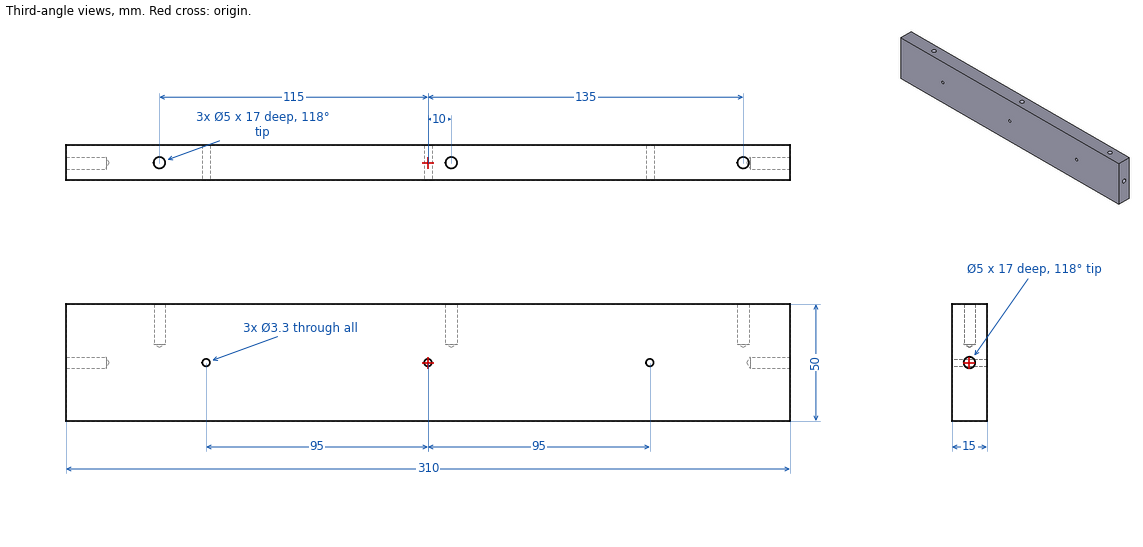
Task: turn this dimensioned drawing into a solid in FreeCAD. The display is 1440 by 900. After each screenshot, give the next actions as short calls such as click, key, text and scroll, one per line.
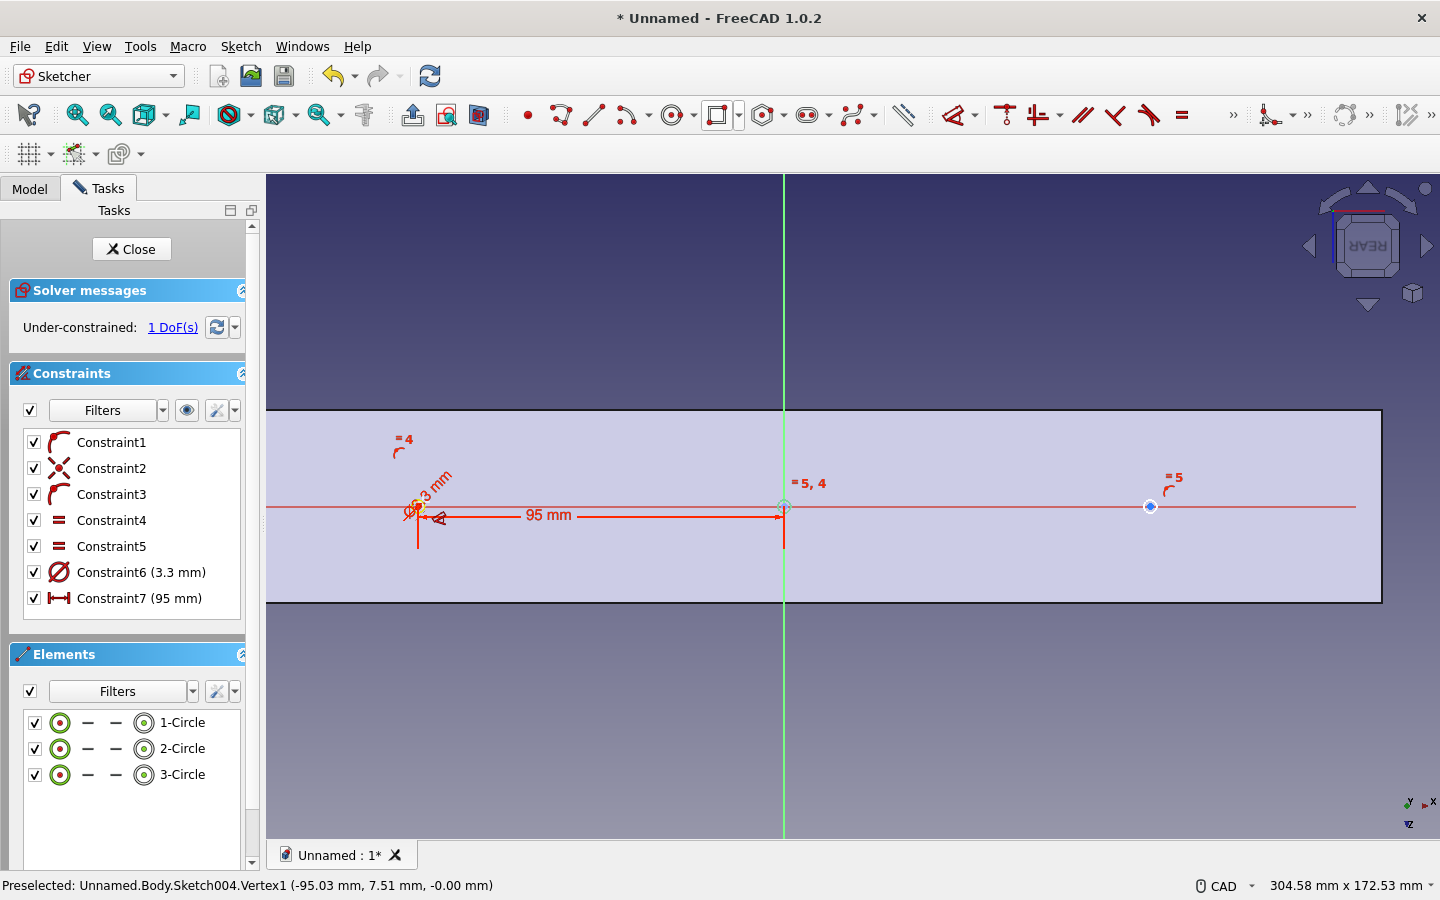
click(1150, 507)
click(967, 541)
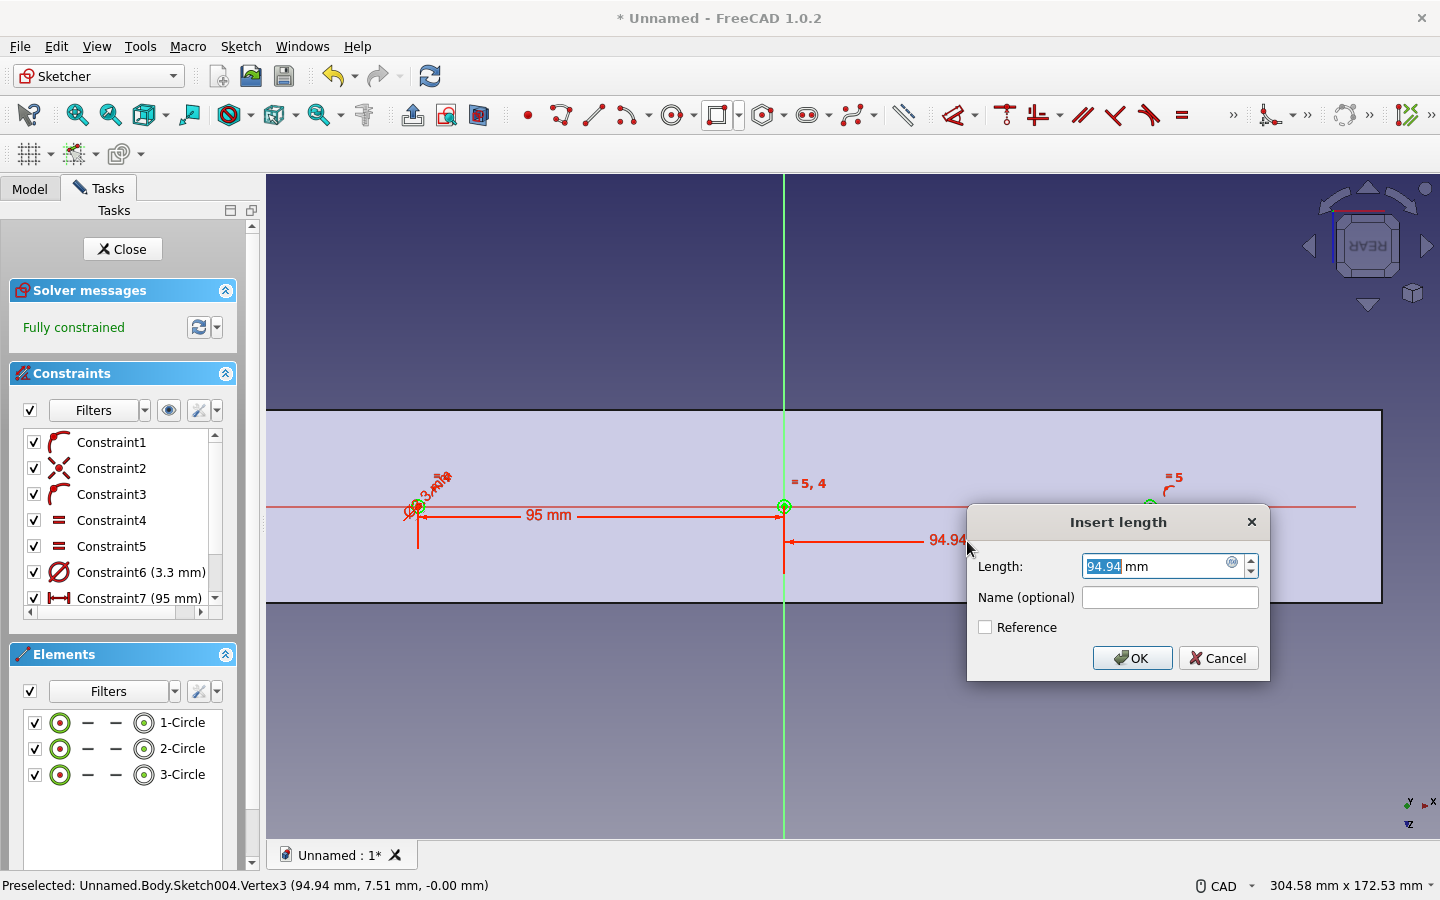
text(95)
key(Return)
key(Escape)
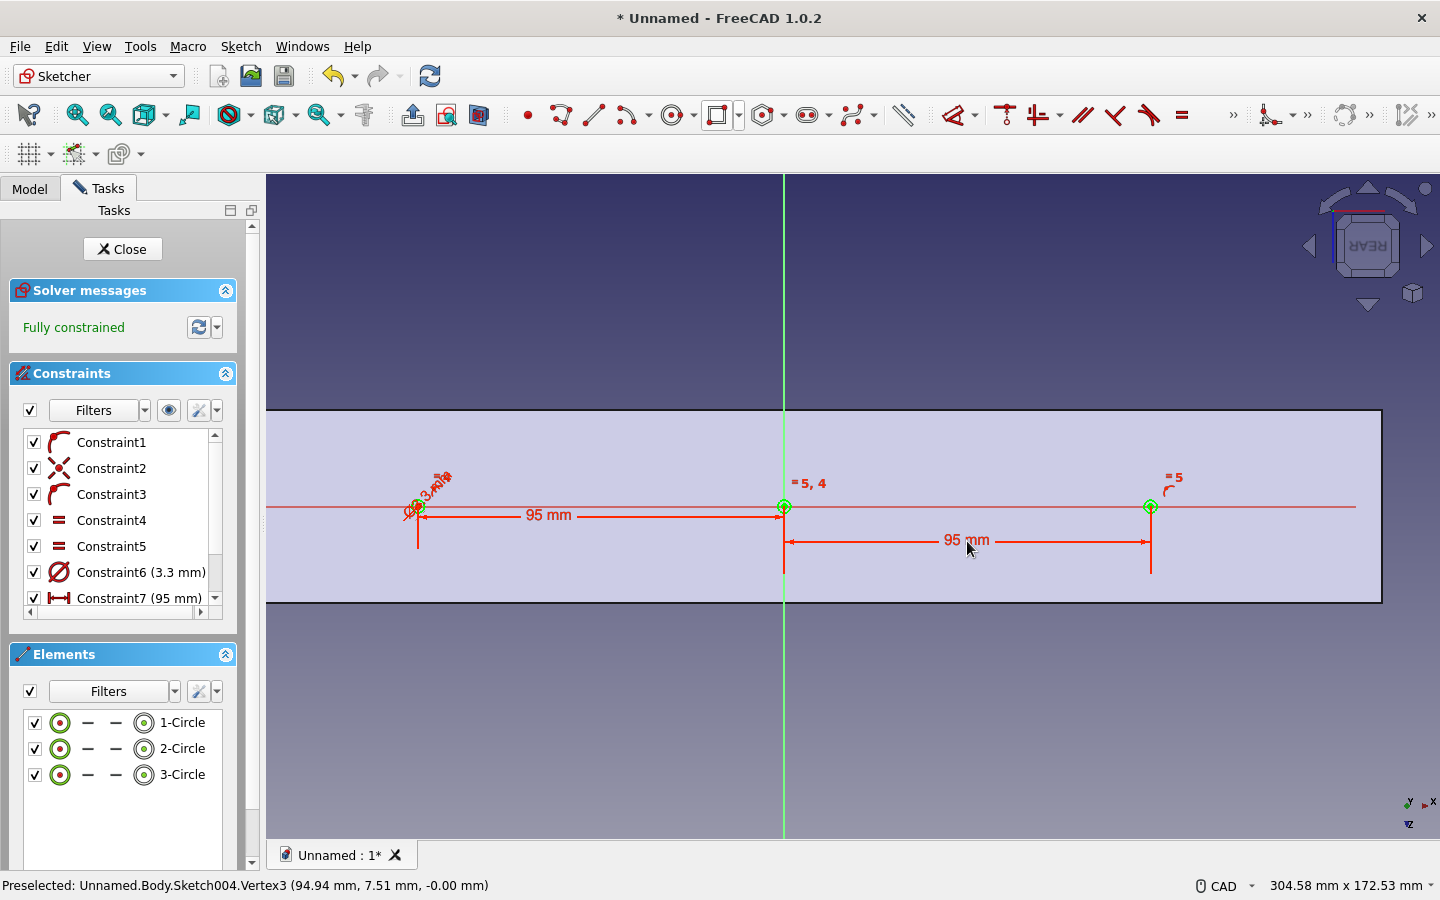
click(123, 249)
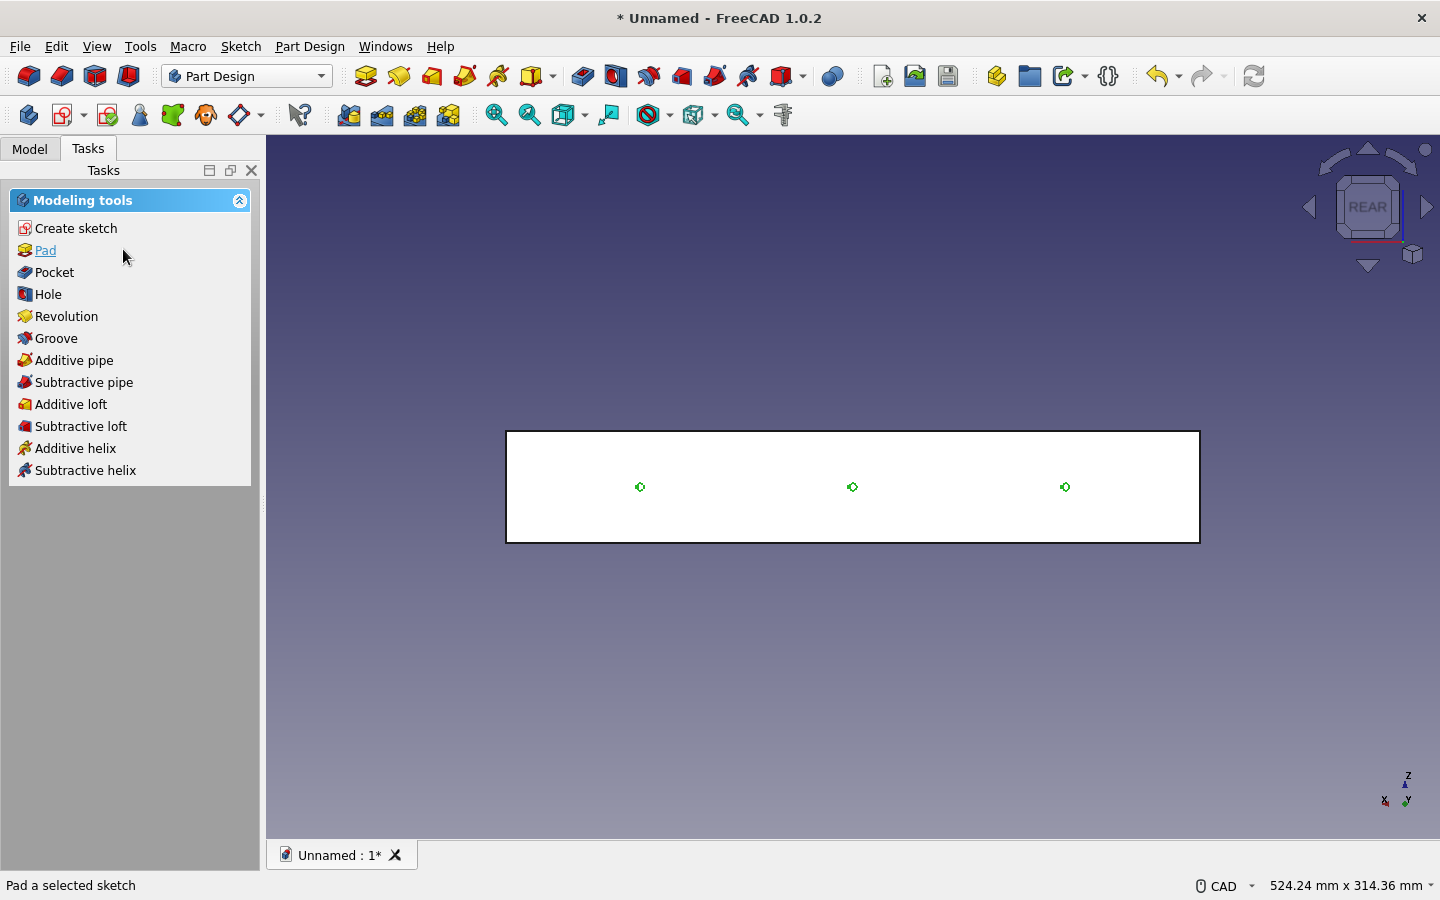
click(616, 76)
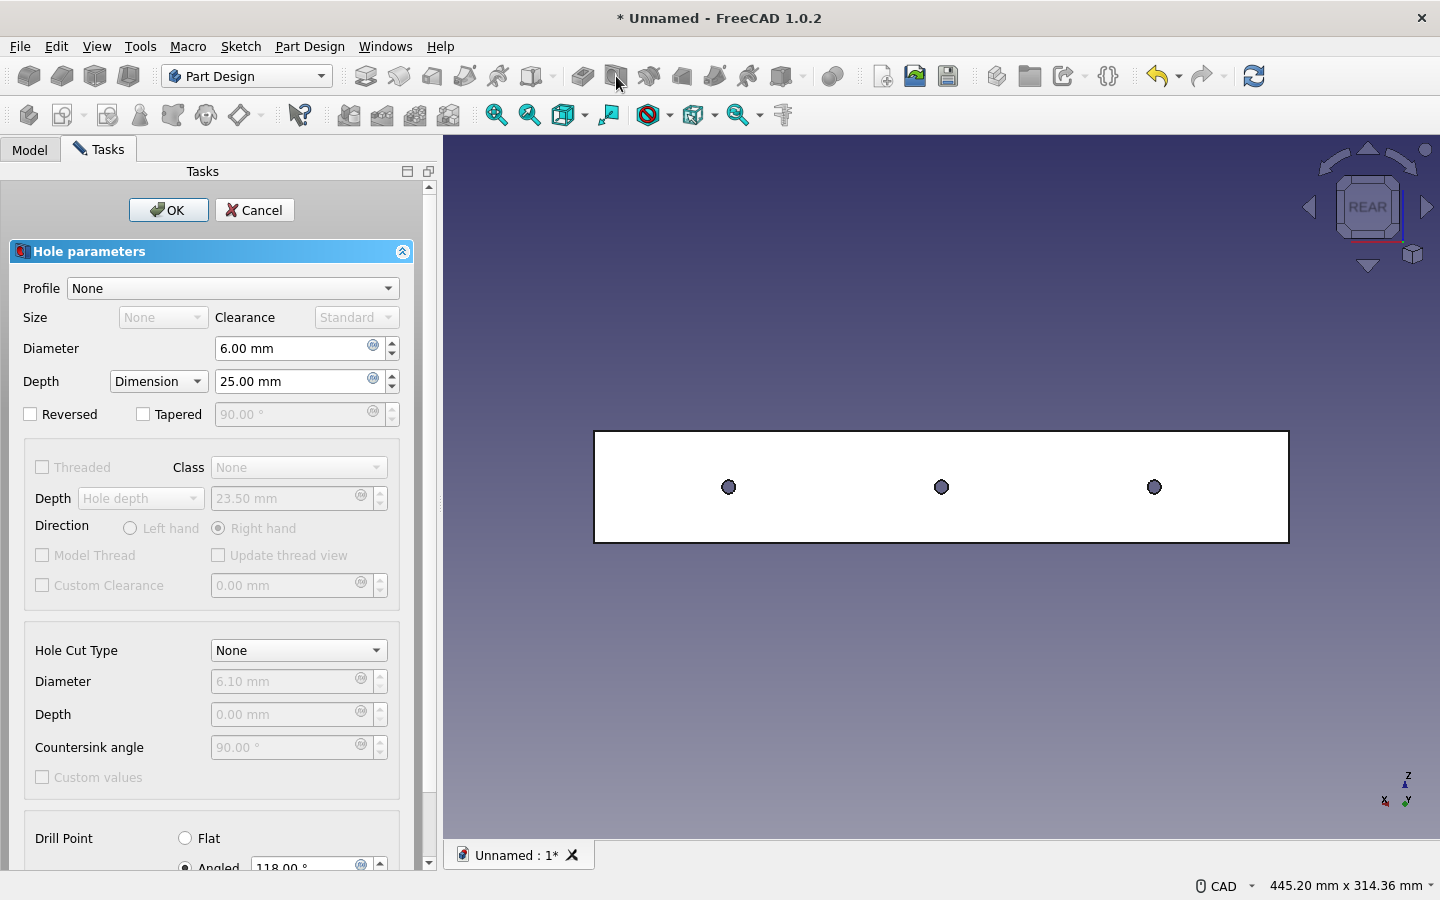
triple_click(300, 348)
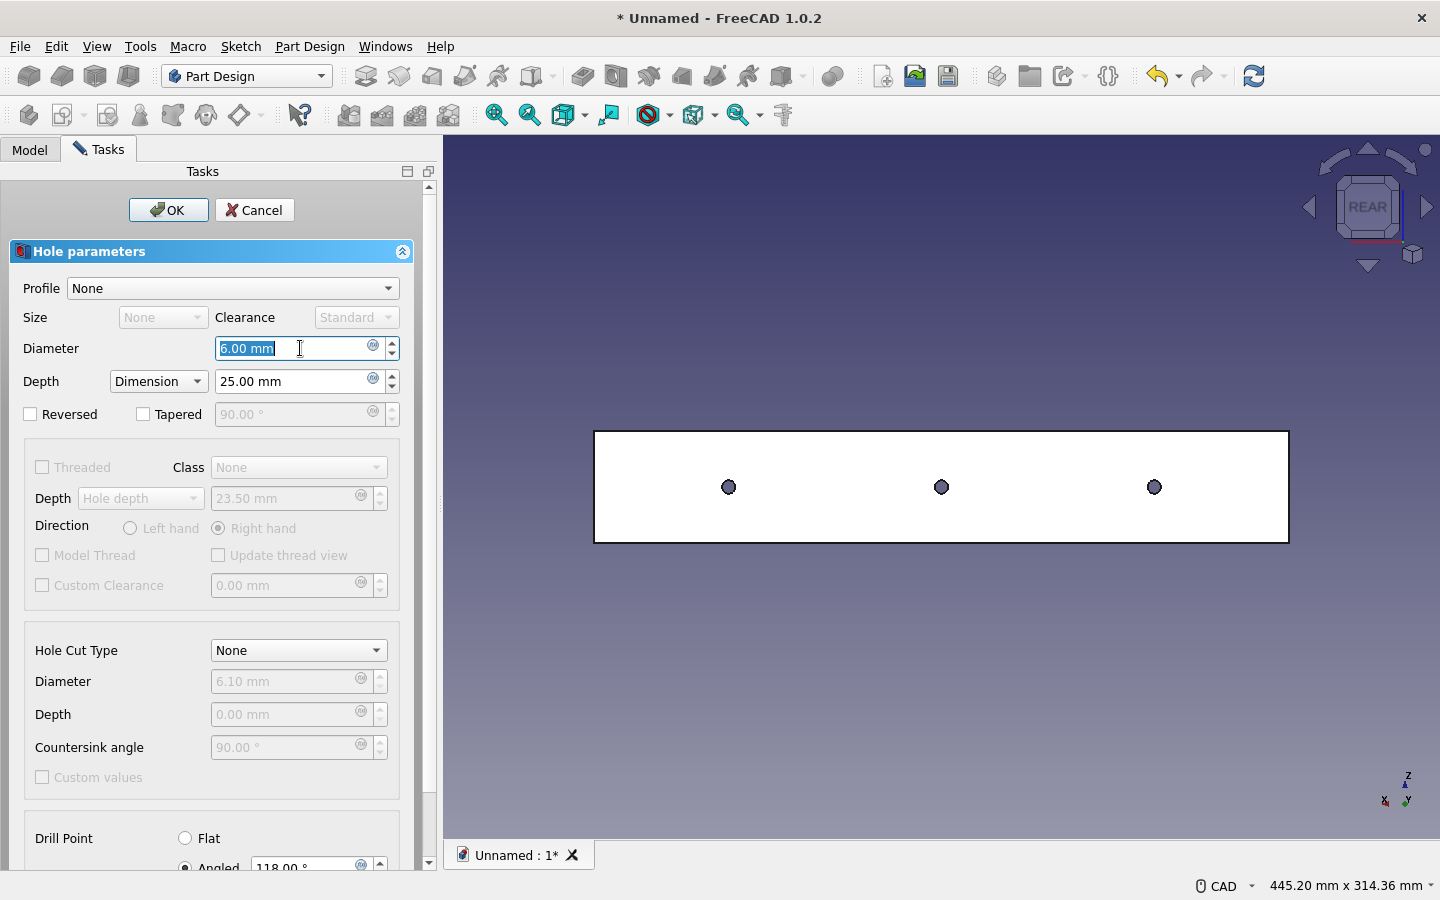
text(3.3)
key(Tab)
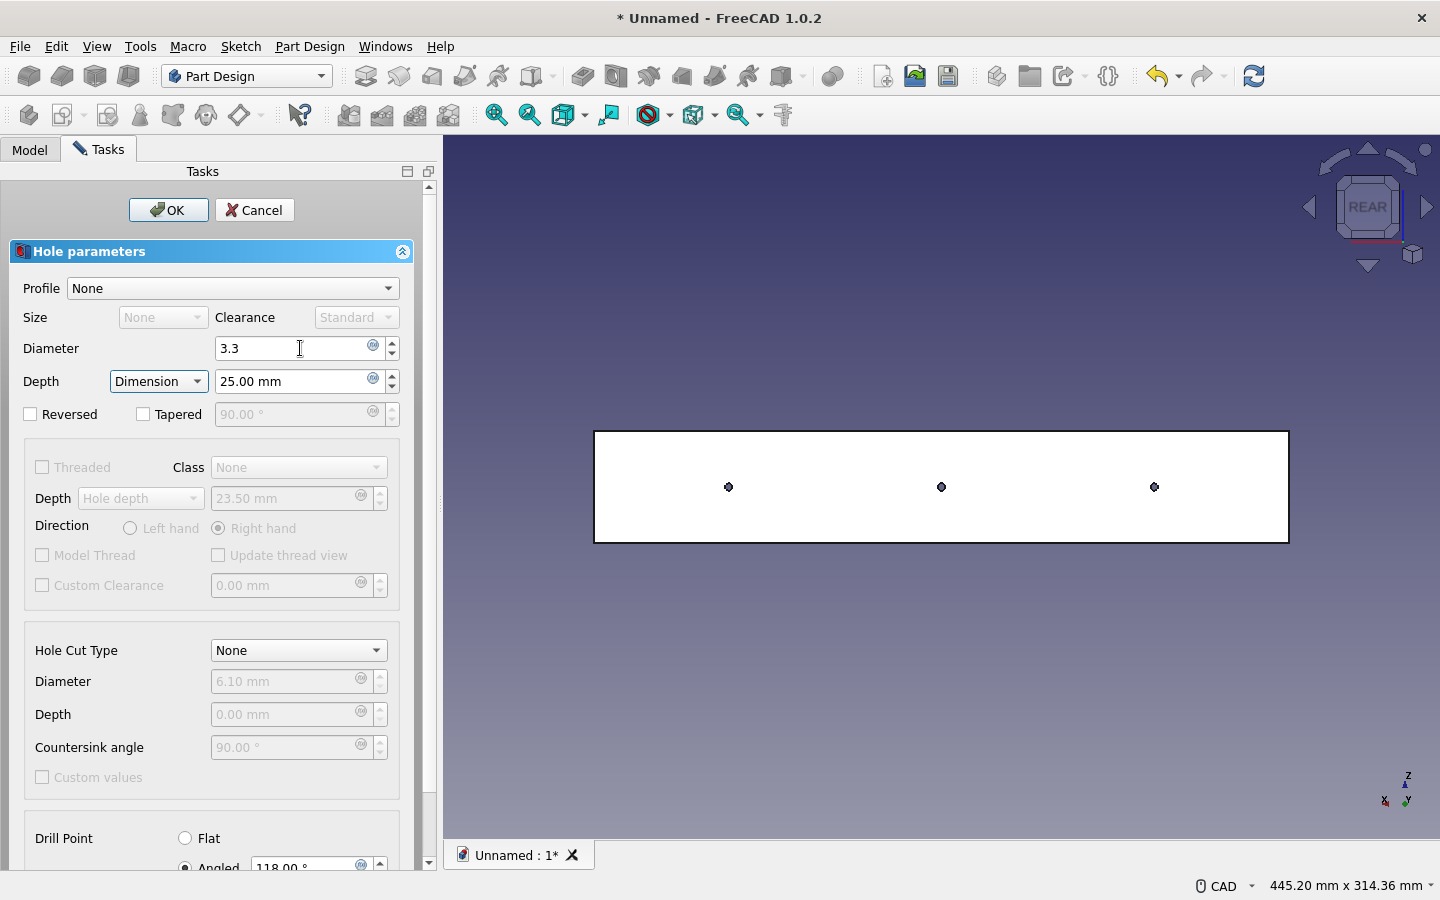
click(160, 382)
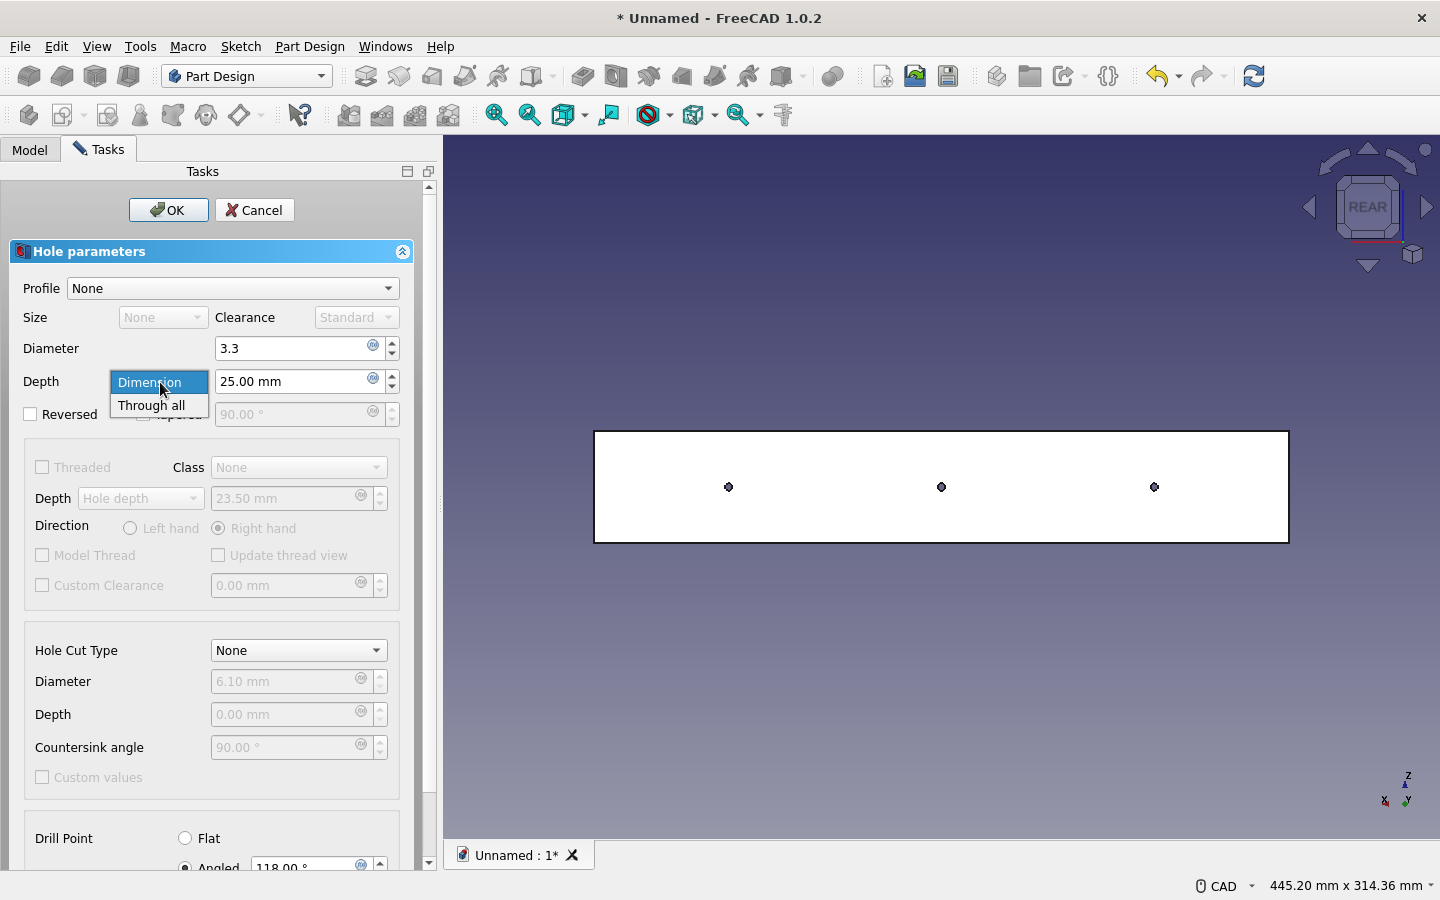
click(158, 406)